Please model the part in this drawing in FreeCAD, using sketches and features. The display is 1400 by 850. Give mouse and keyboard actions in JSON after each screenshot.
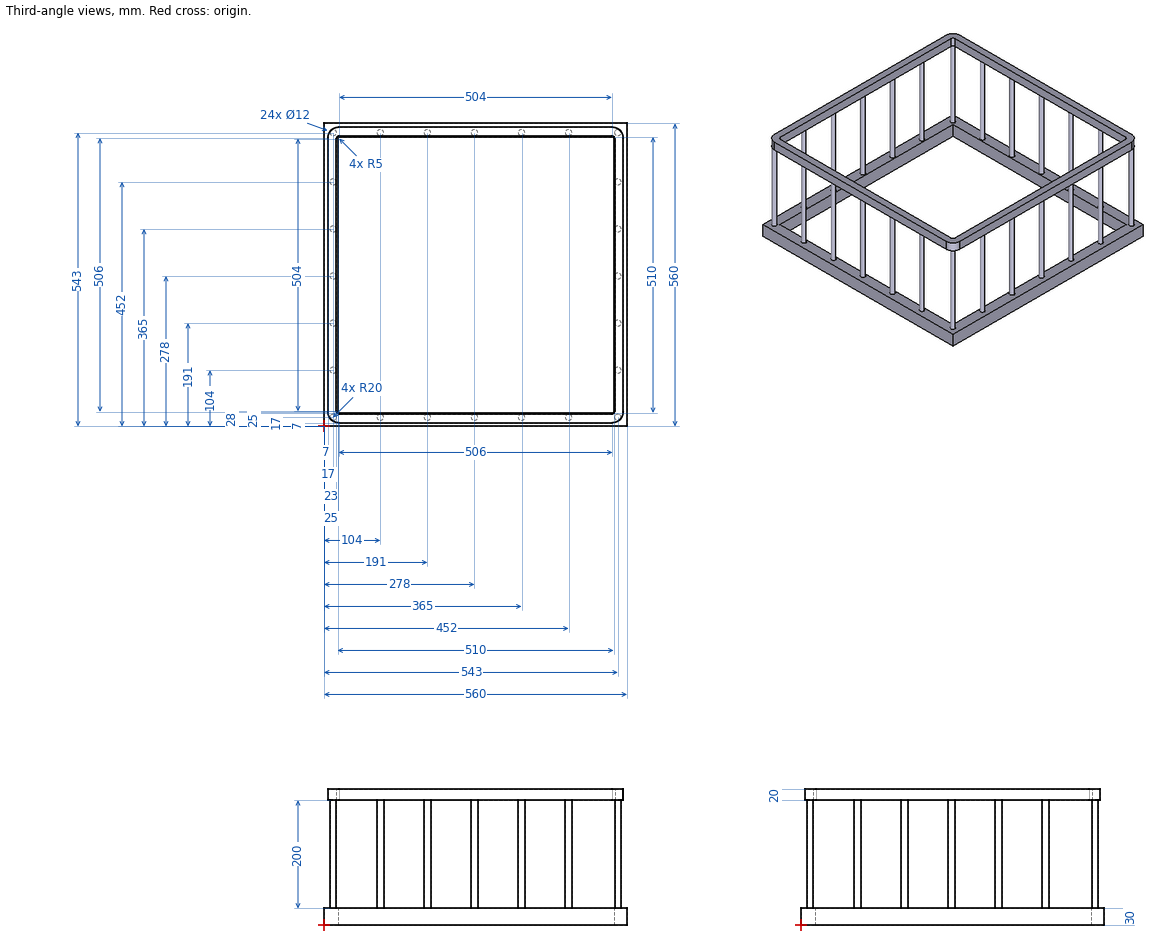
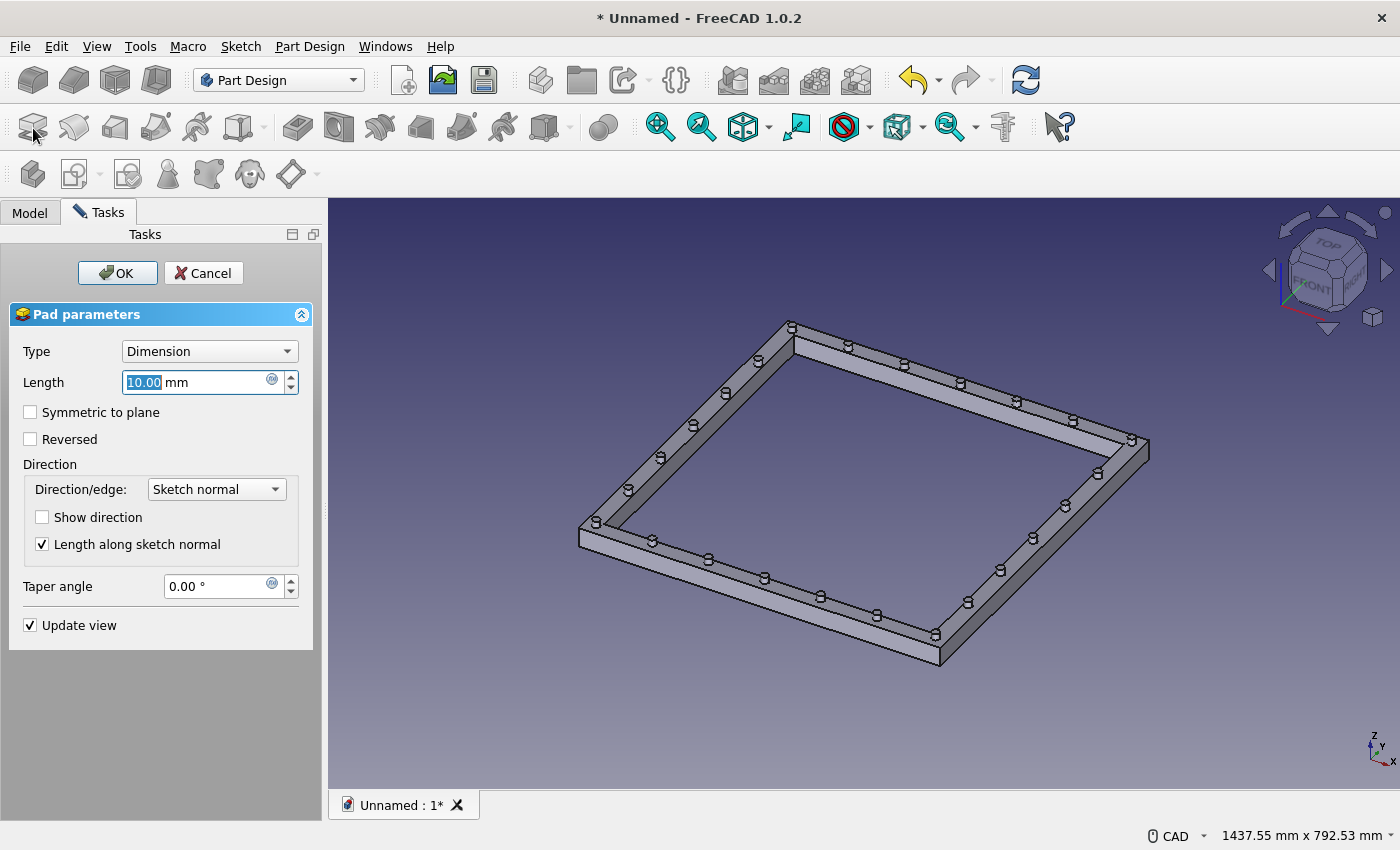
{"action": "type", "text": "200"}
{"action": "key", "text": "Tab"}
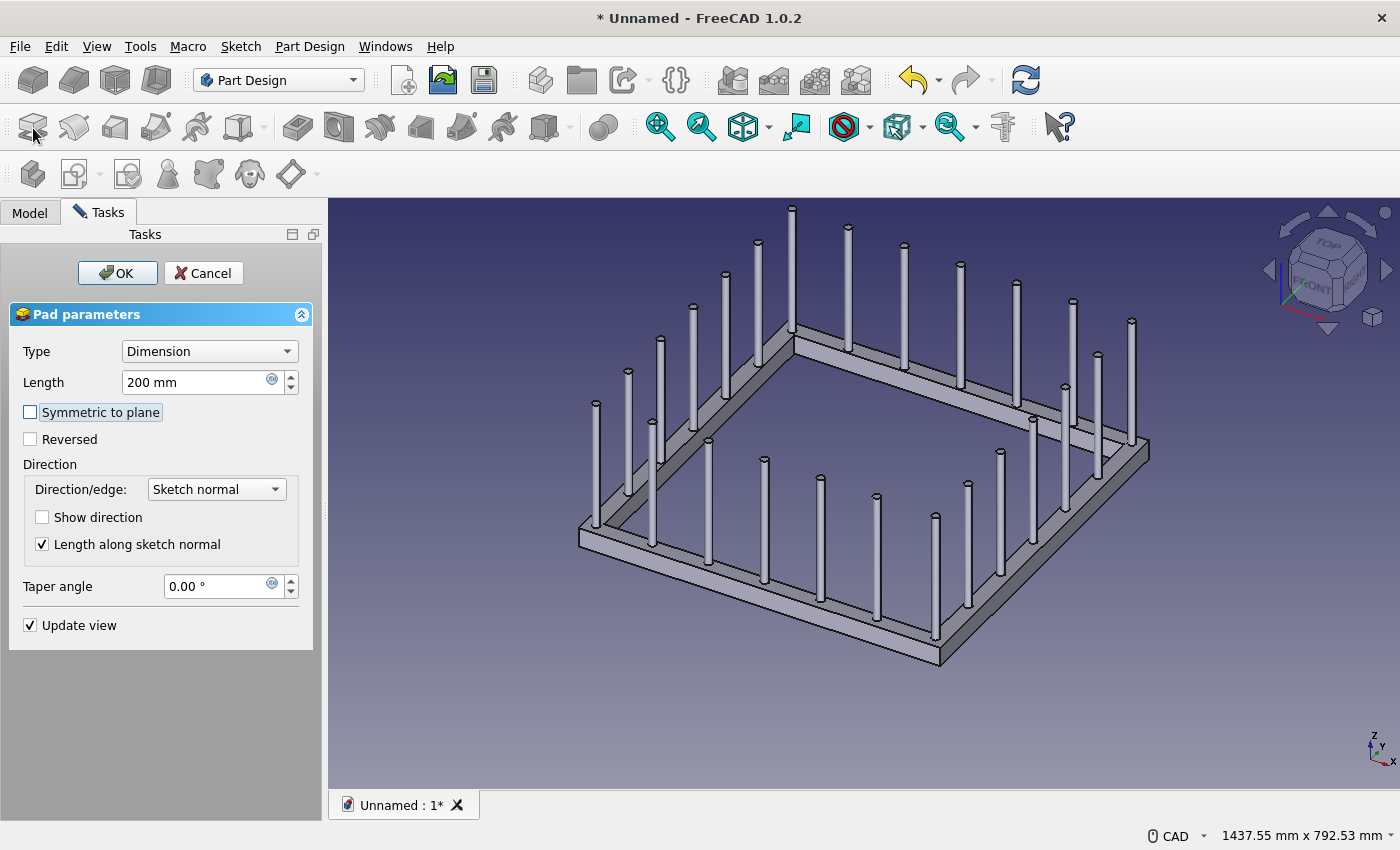
{"action": "left_click", "coordinate": [118, 273]}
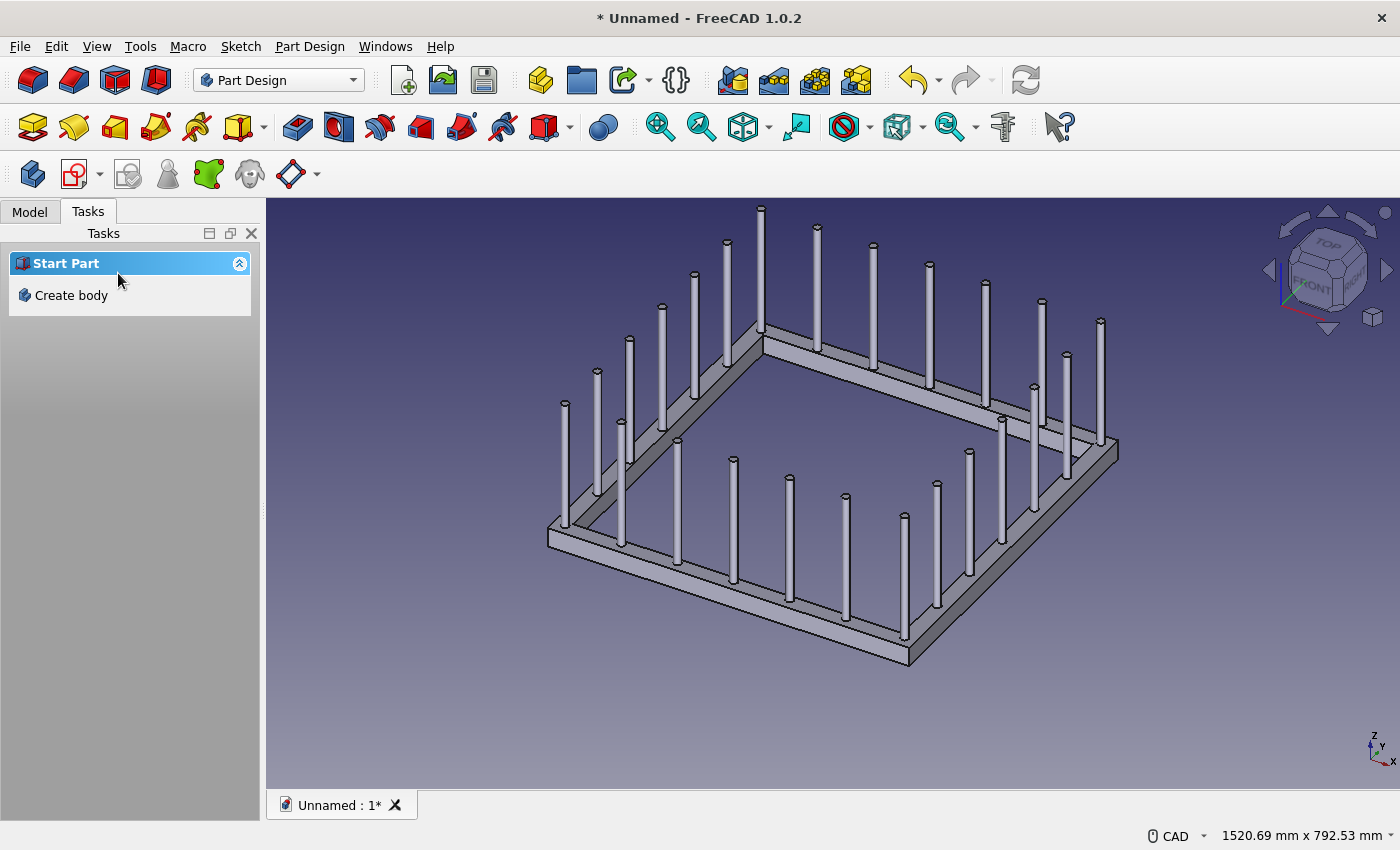
{"action": "scroll", "coordinate": [930, 263], "scroll_direction": "up", "scroll_amount": 5}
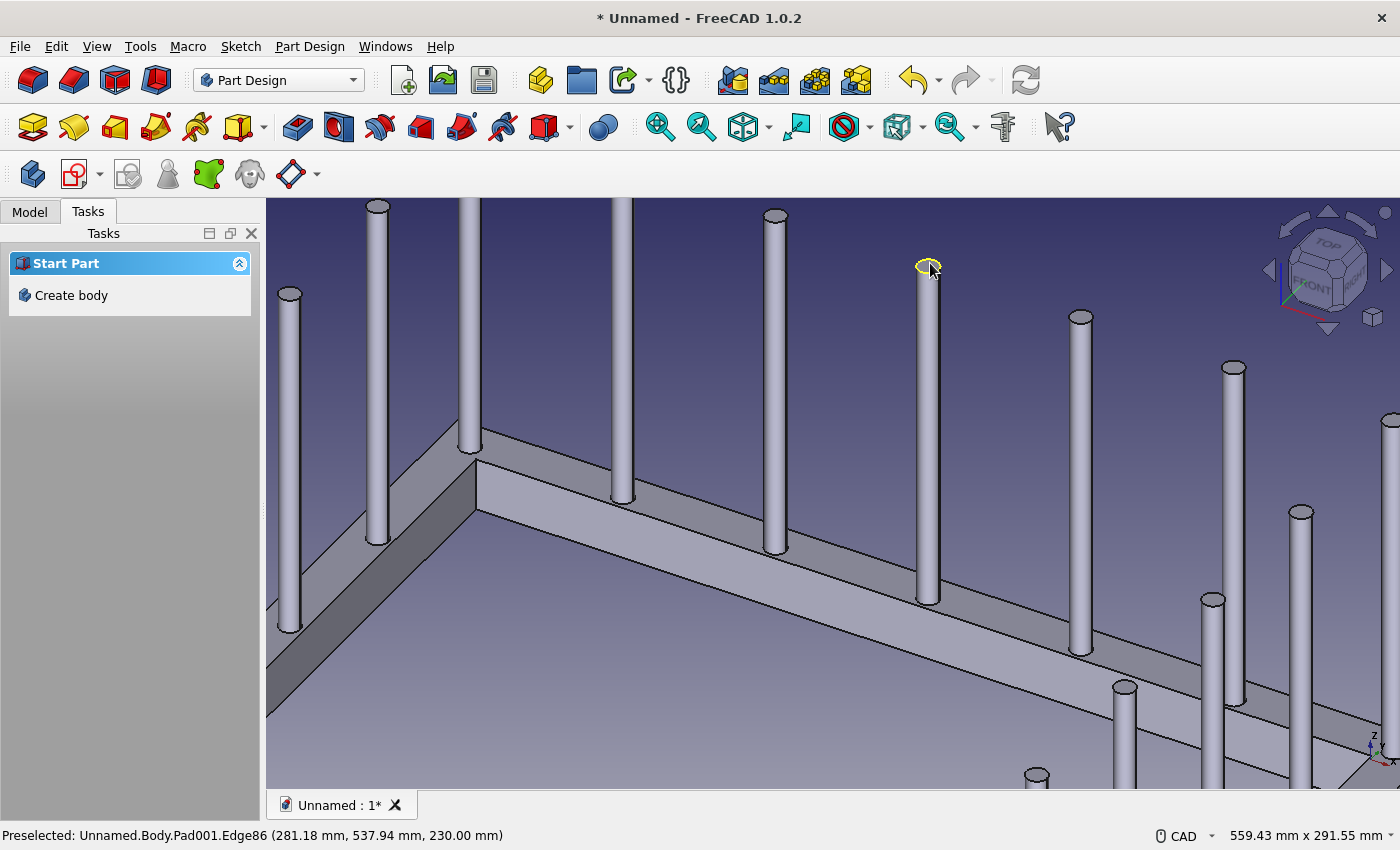
{"action": "left_click", "coordinate": [927, 263]}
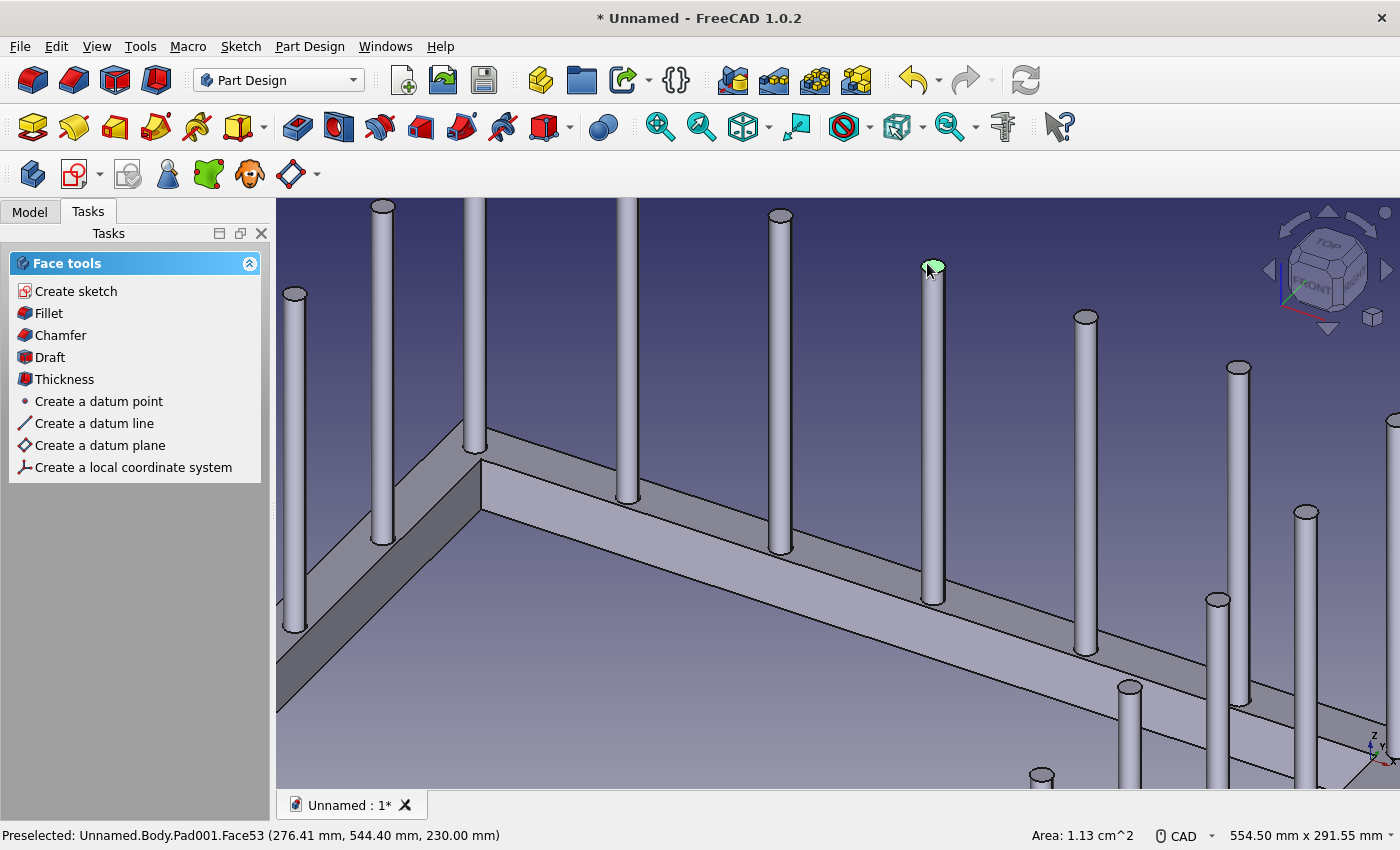
{"action": "left_click", "coordinate": [74, 174]}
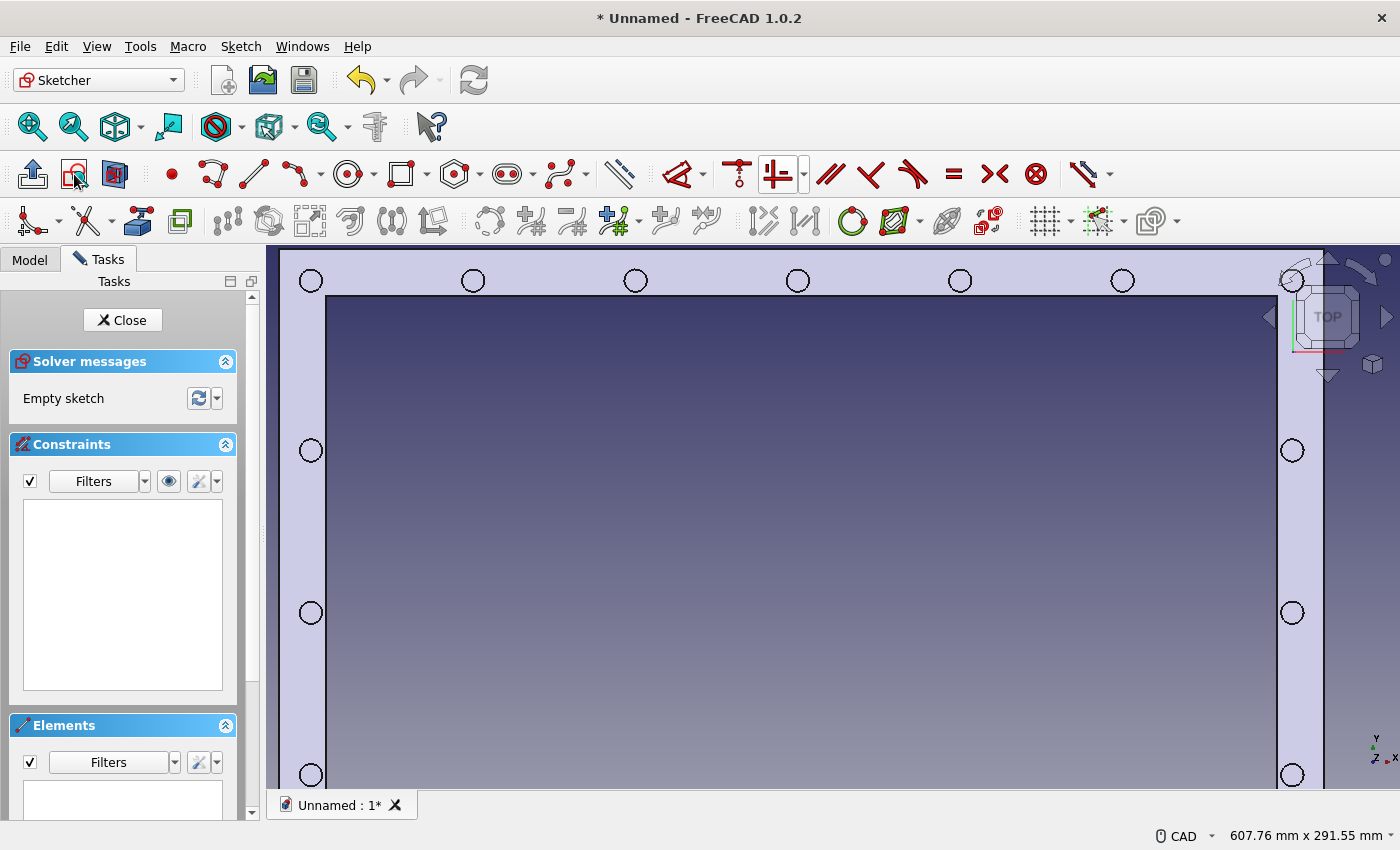
{"action": "scroll", "coordinate": [747, 365], "scroll_direction": "down", "scroll_amount": 5}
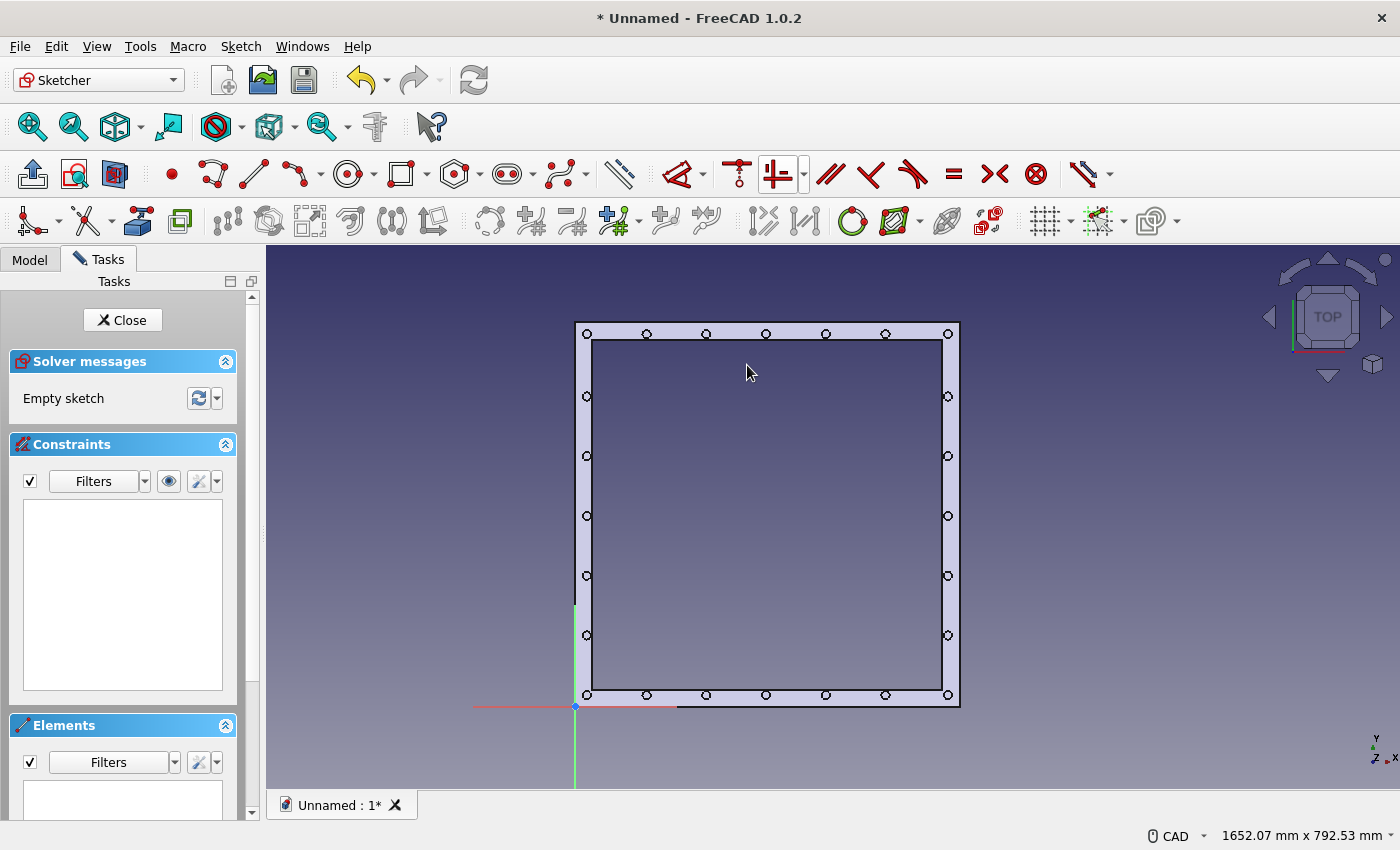
{"action": "left_click", "coordinate": [254, 174]}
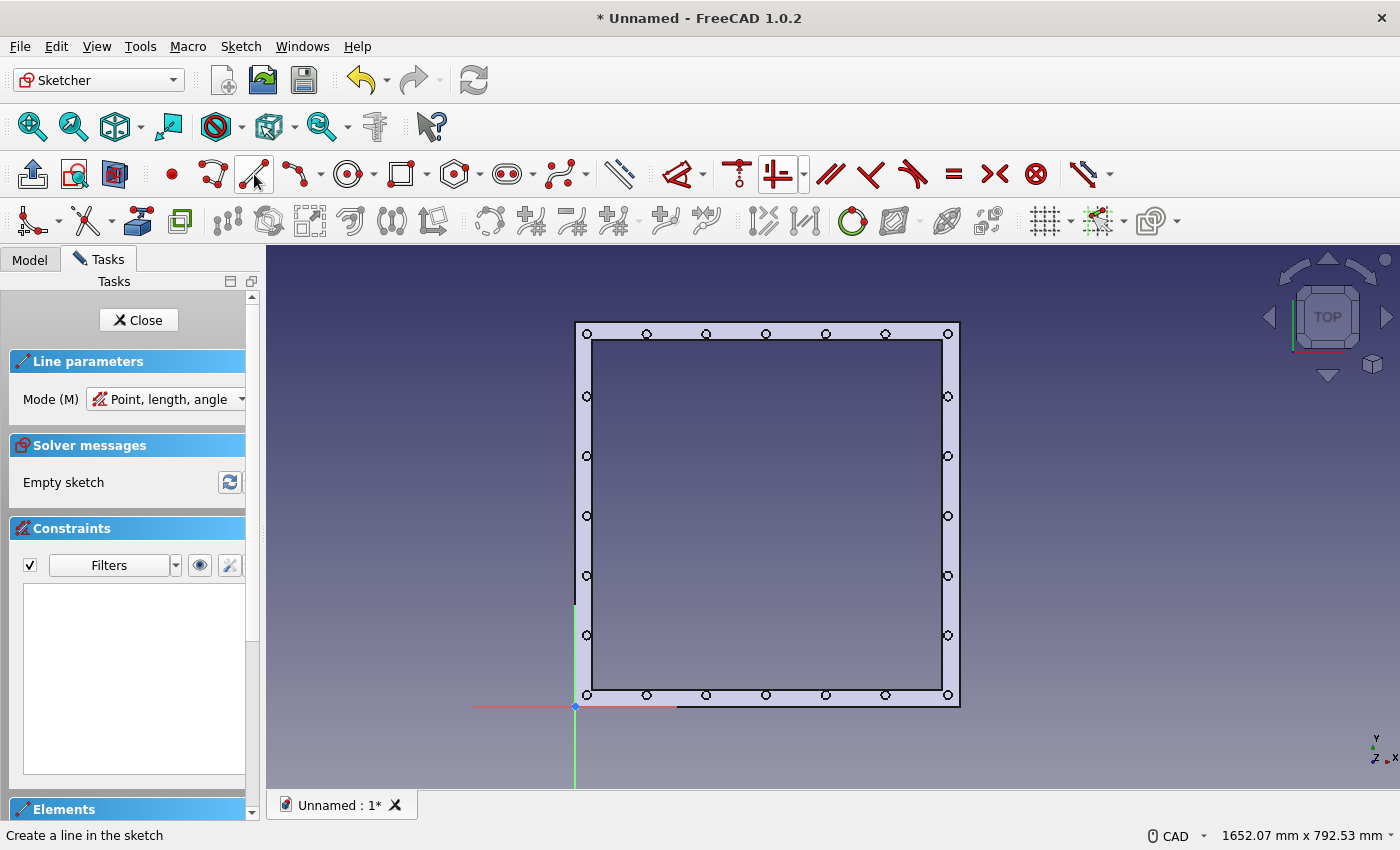
{"action": "scroll", "coordinate": [580, 341], "scroll_direction": "up", "scroll_amount": 6}